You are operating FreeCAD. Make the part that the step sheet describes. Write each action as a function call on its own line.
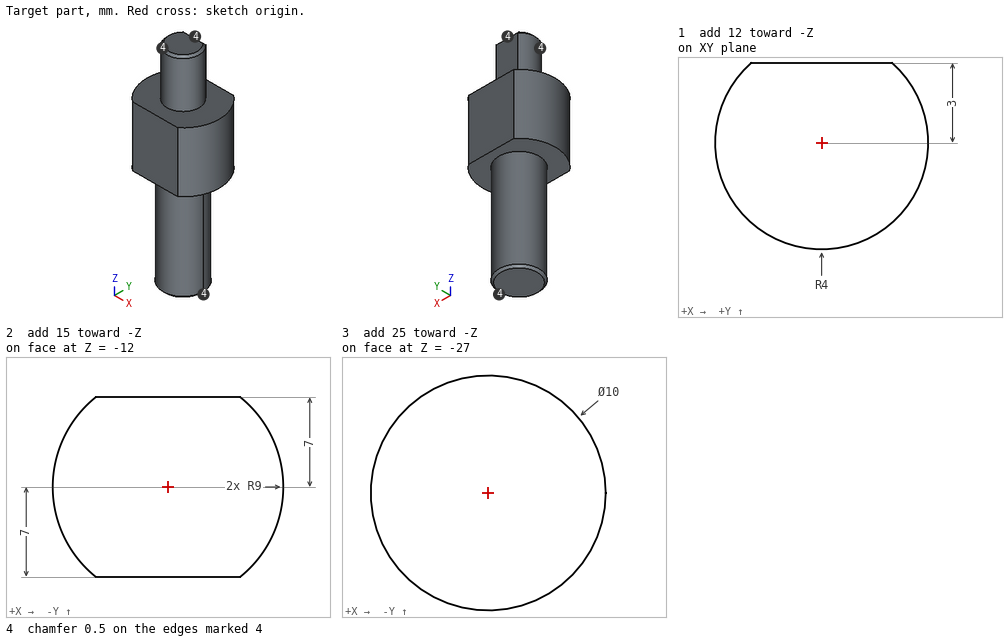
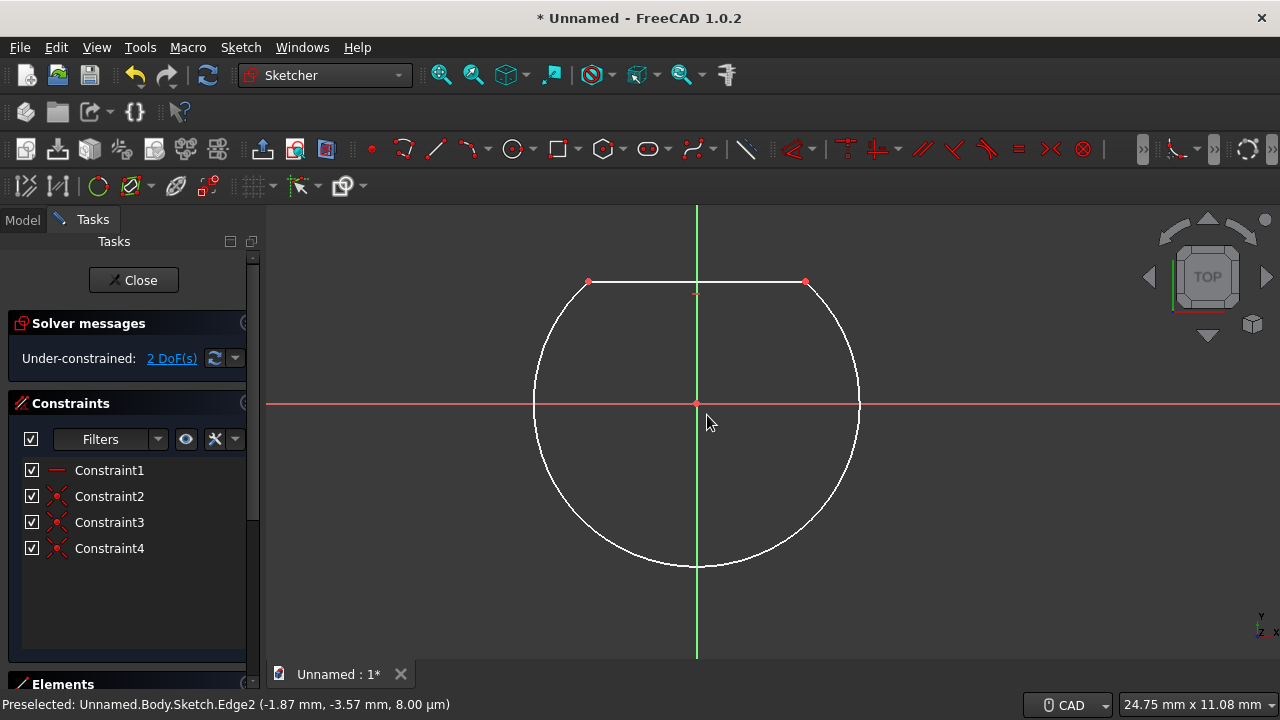
click(792, 150)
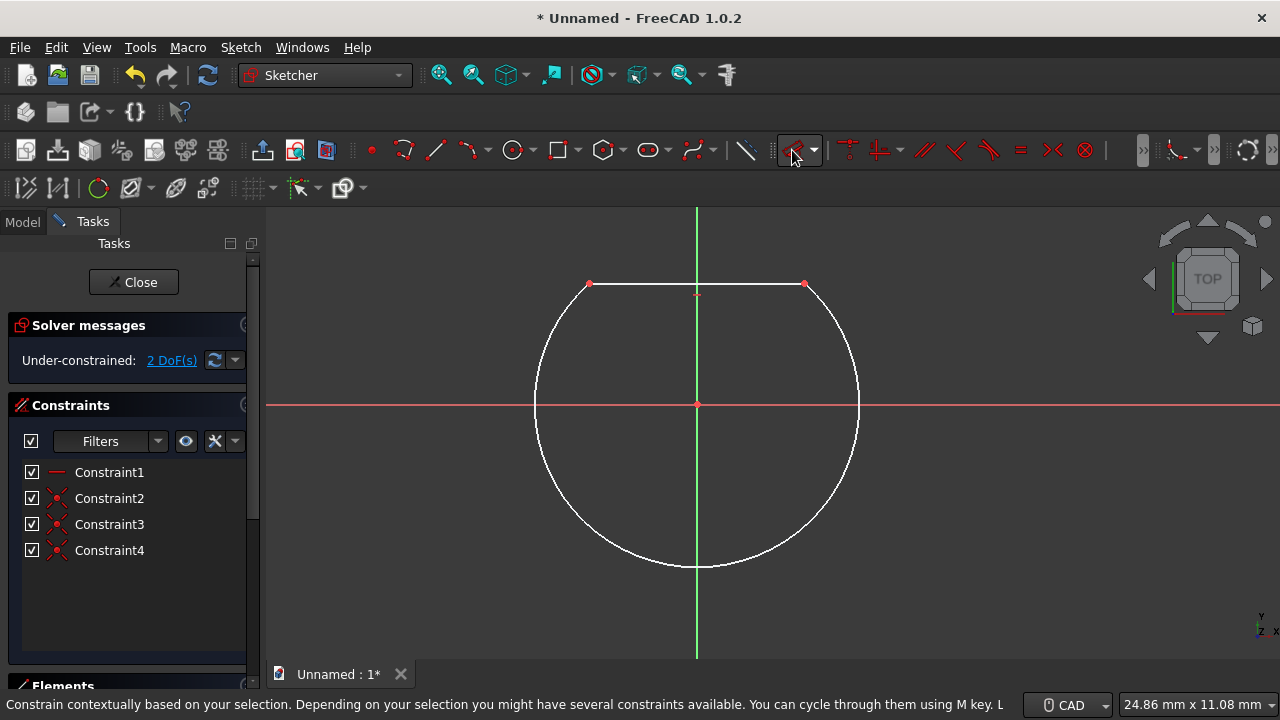
click(564, 497)
click(538, 515)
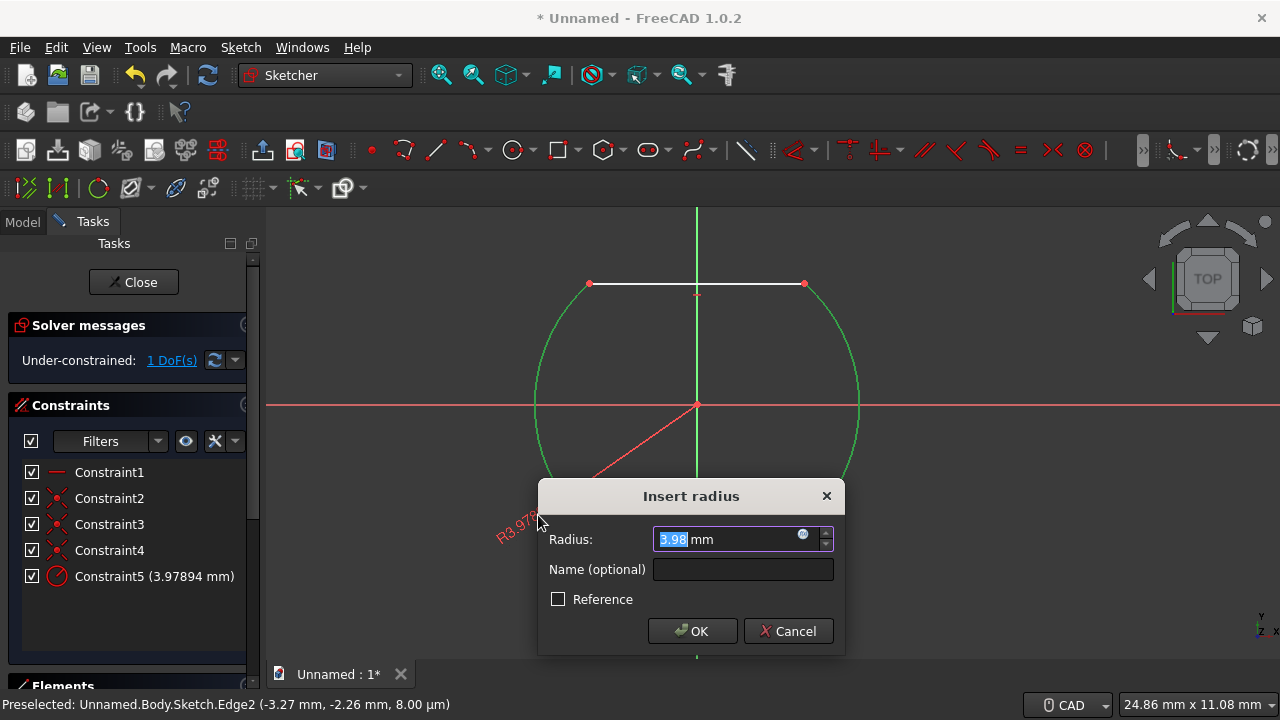
text(4)
key(Return)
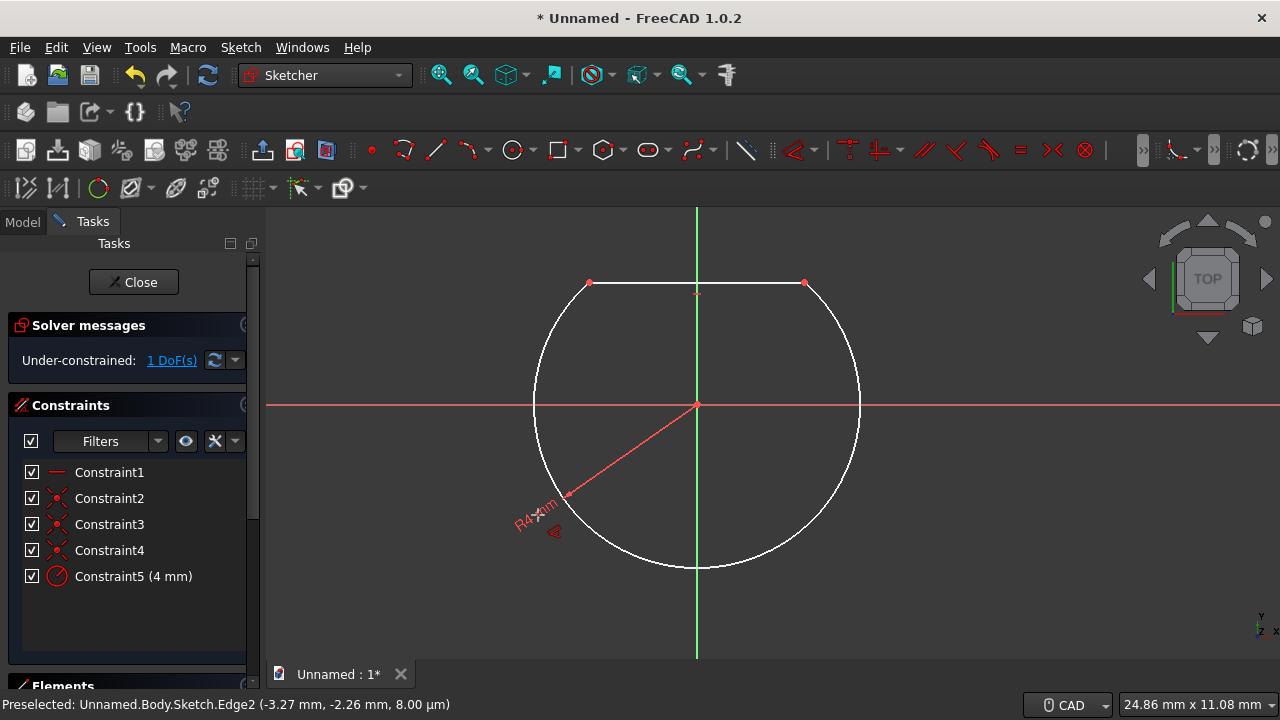
click(805, 283)
click(839, 372)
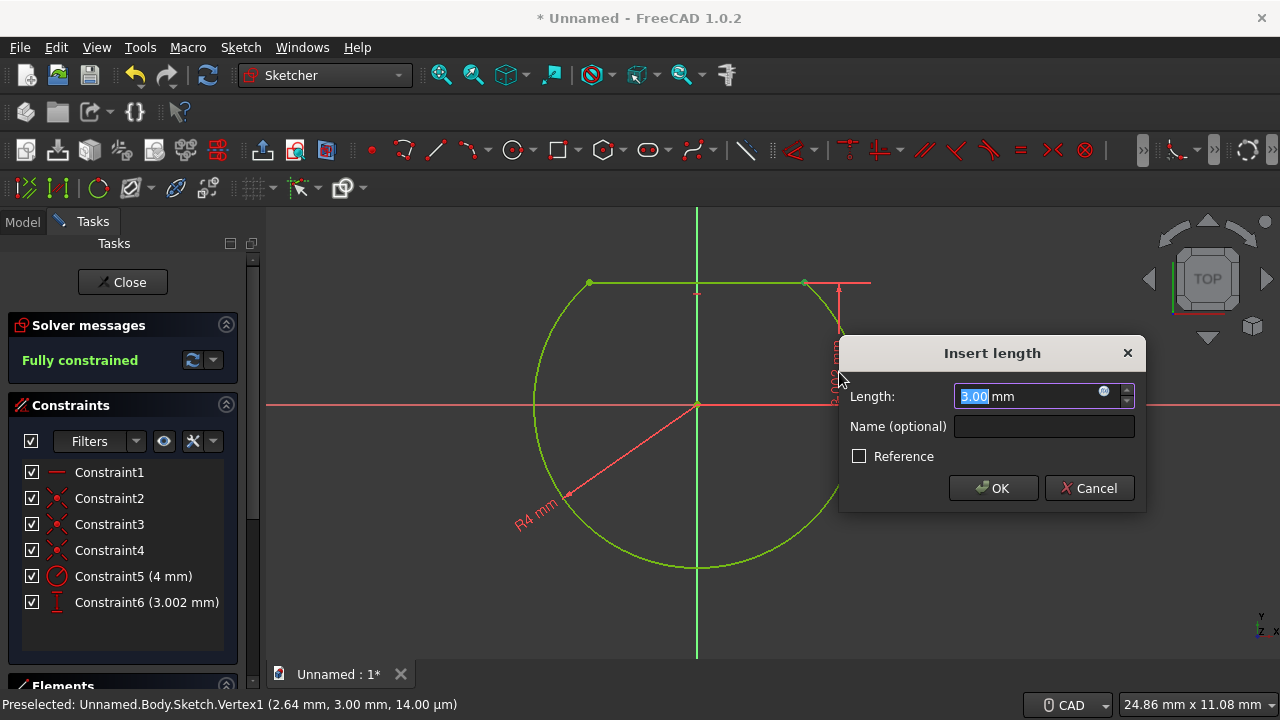
text(3)
key(Return)
key(Escape)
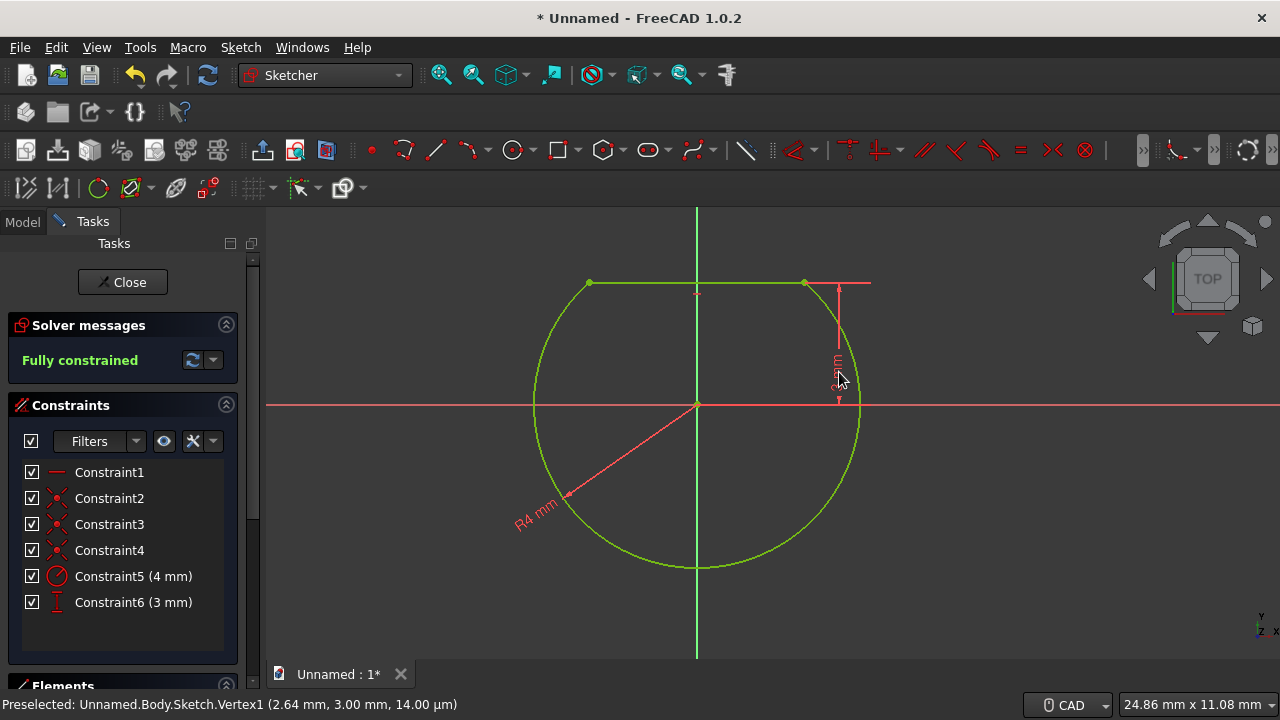
click(123, 282)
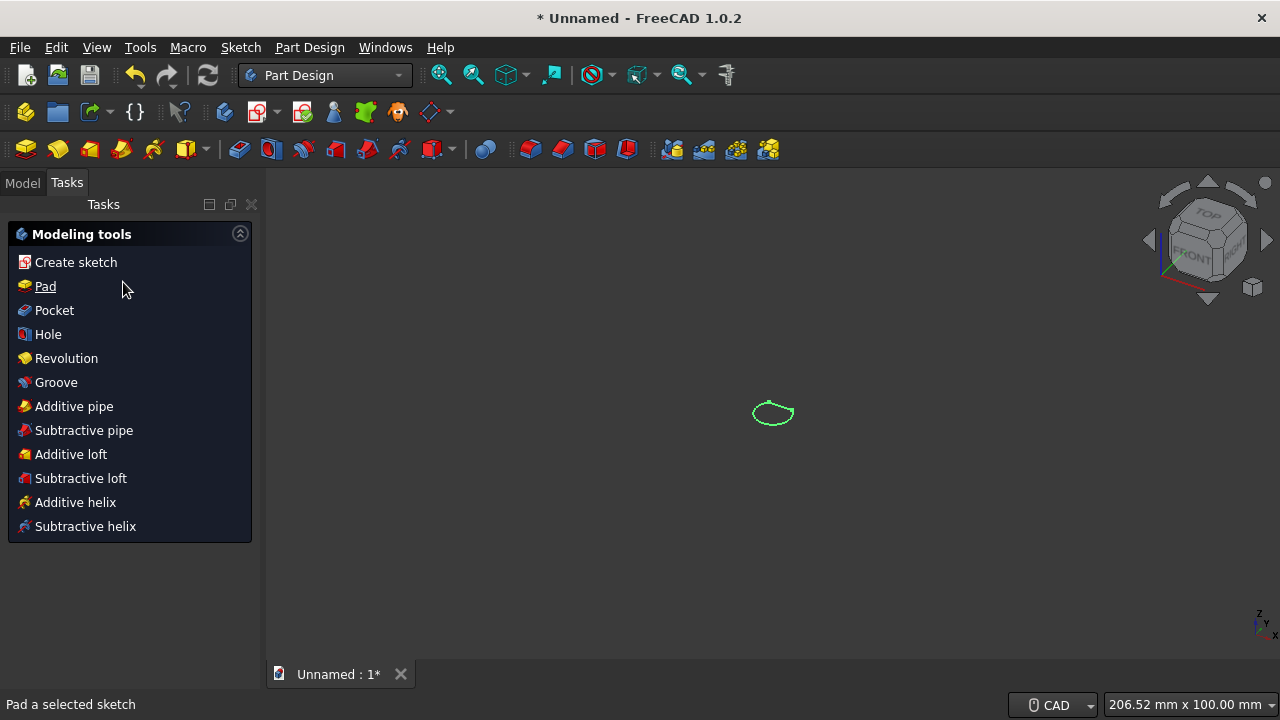
click(26, 150)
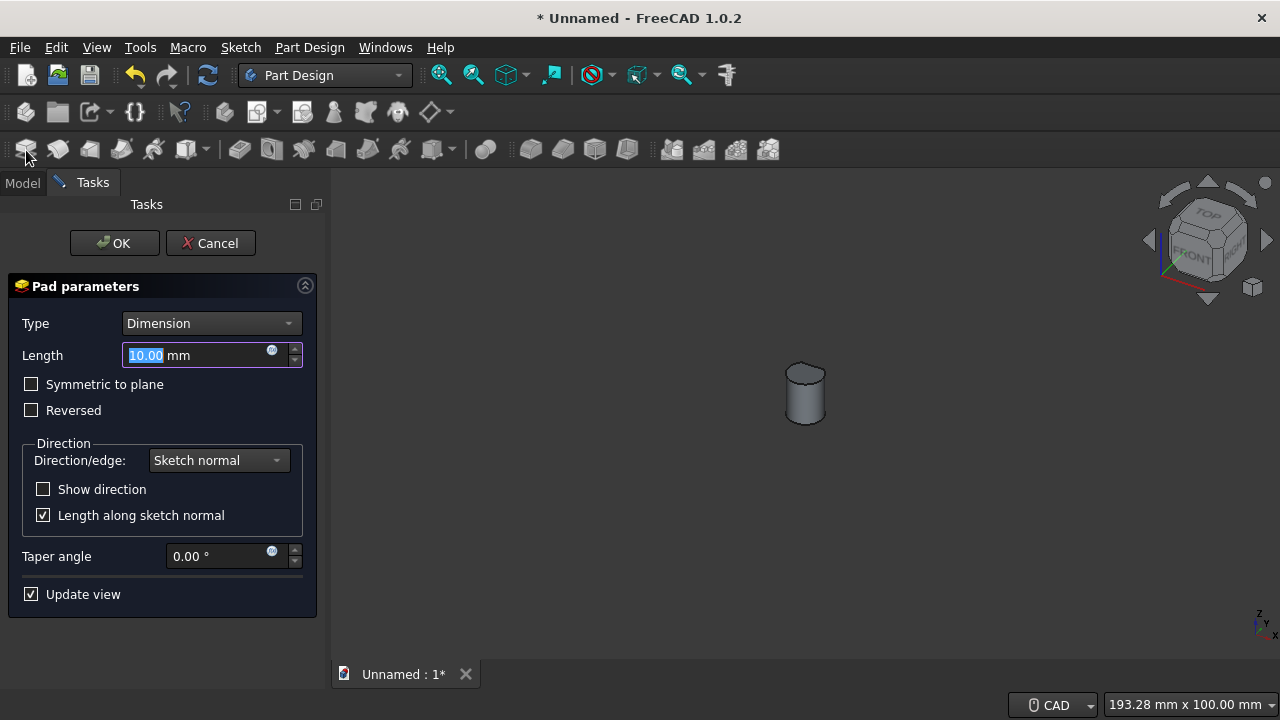
text(12)
key(Tab)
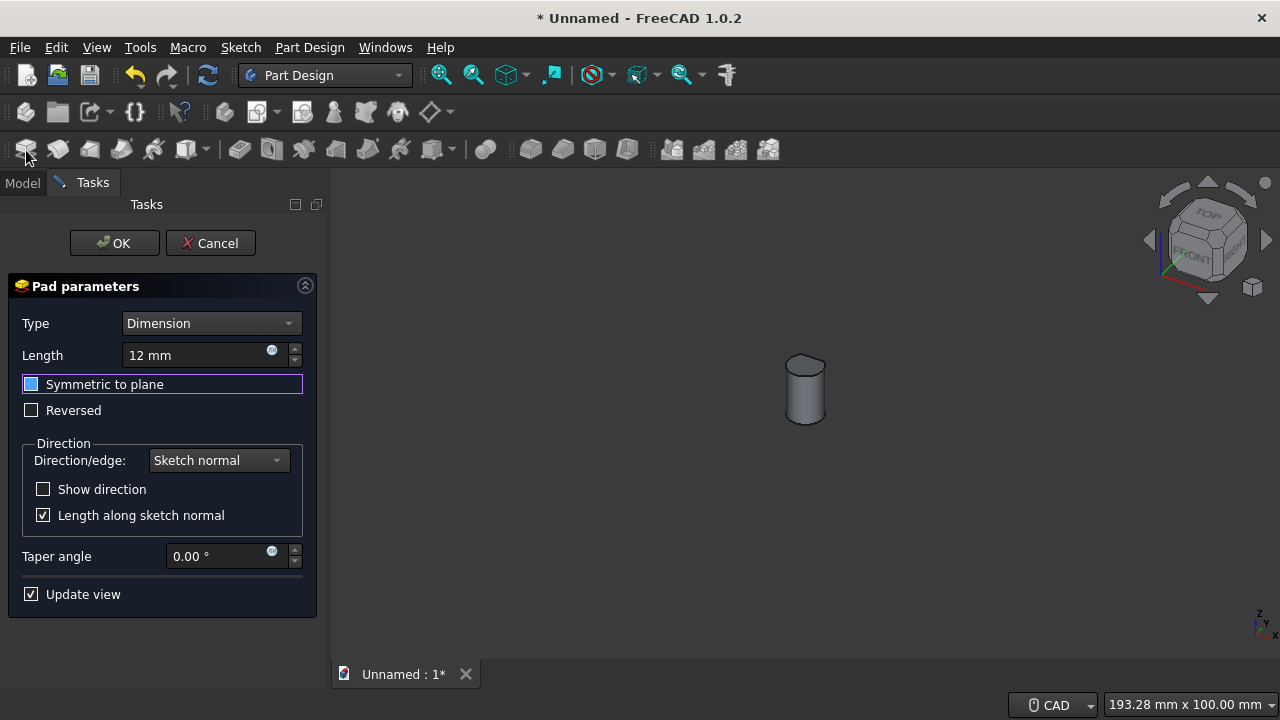
click(30, 410)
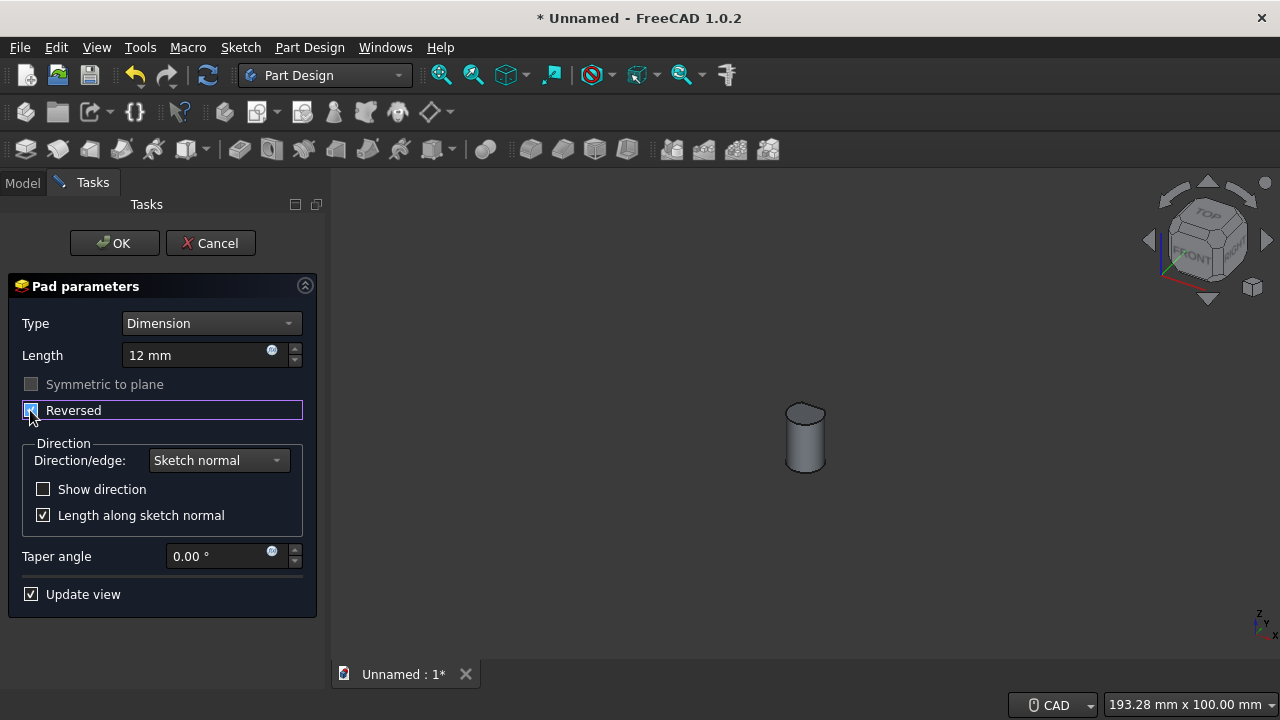
click(115, 243)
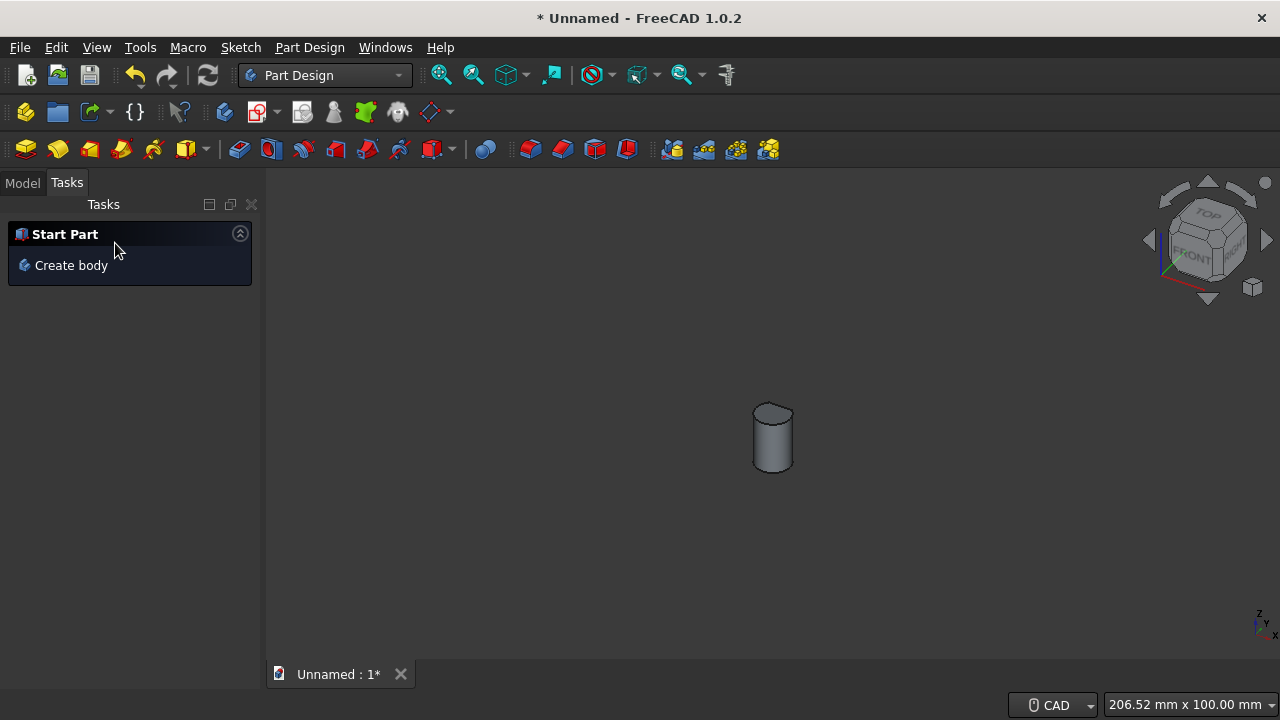
click(442, 76)